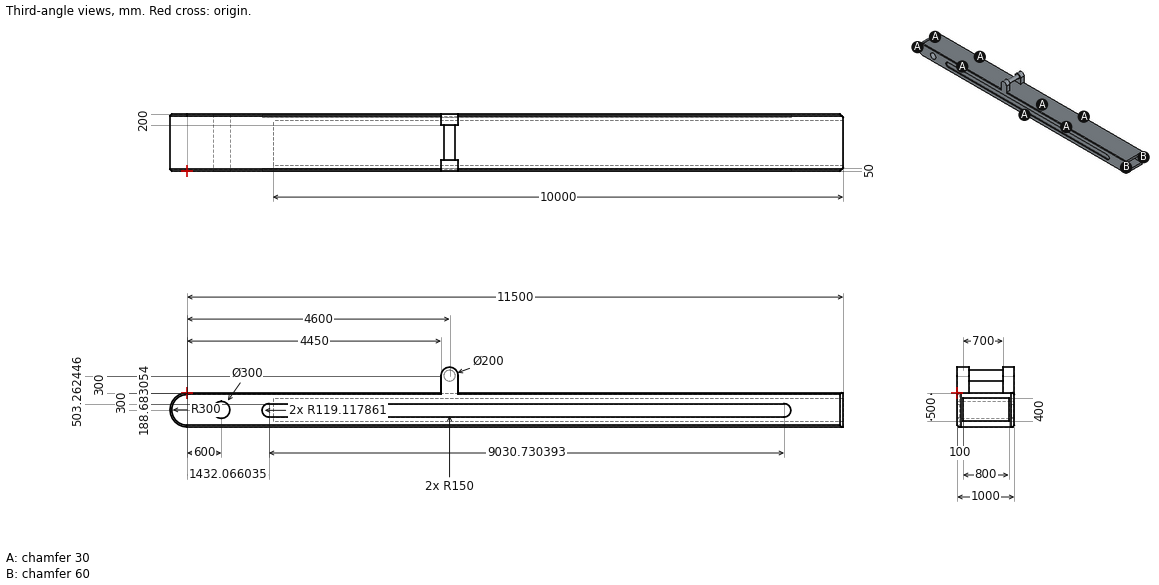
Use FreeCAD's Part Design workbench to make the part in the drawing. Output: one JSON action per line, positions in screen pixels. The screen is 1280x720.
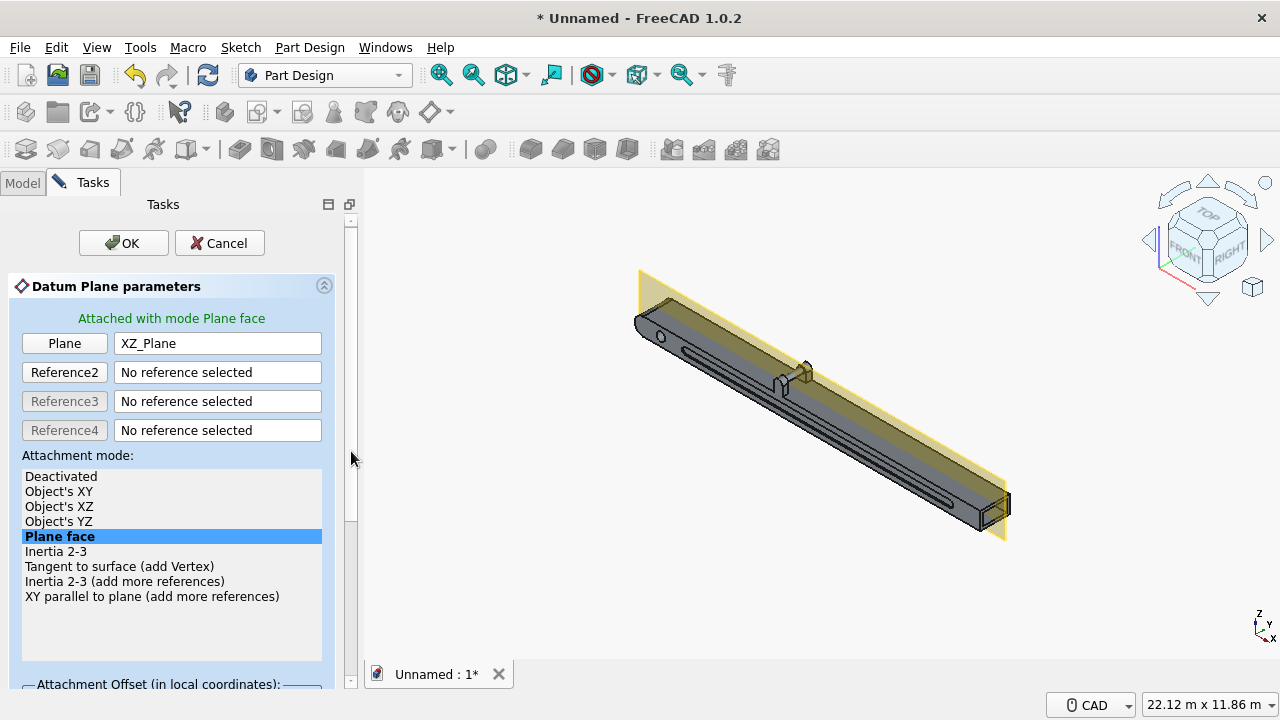
{"action": "left_click", "coordinate": [124, 243]}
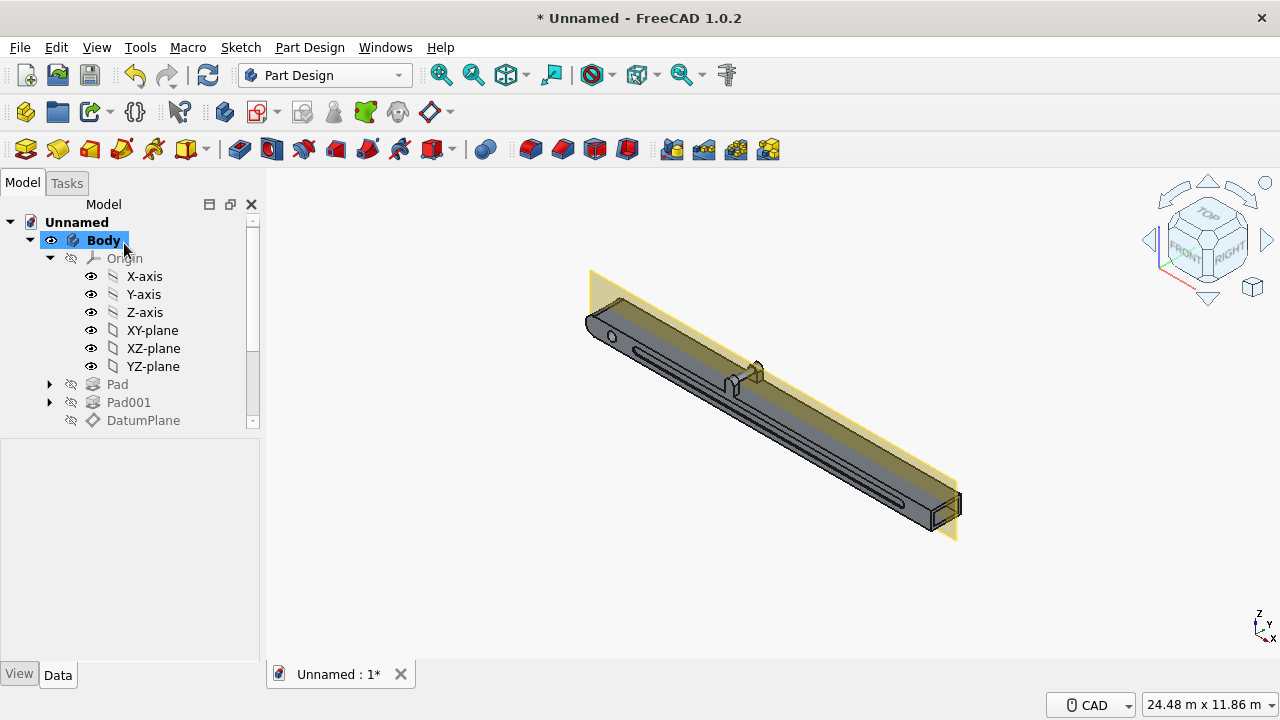
{"action": "scroll", "coordinate": [100, 326], "scroll_direction": "down", "scroll_amount": 3}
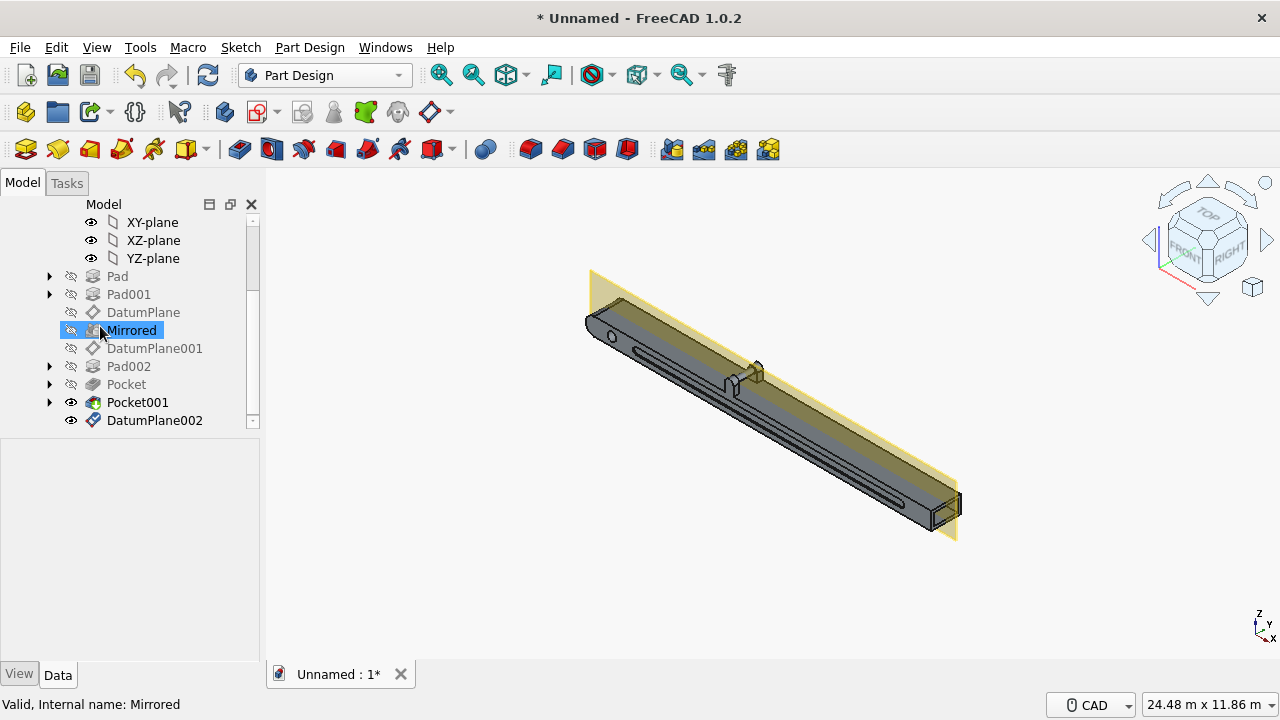
{"action": "left_click", "coordinate": [116, 402]}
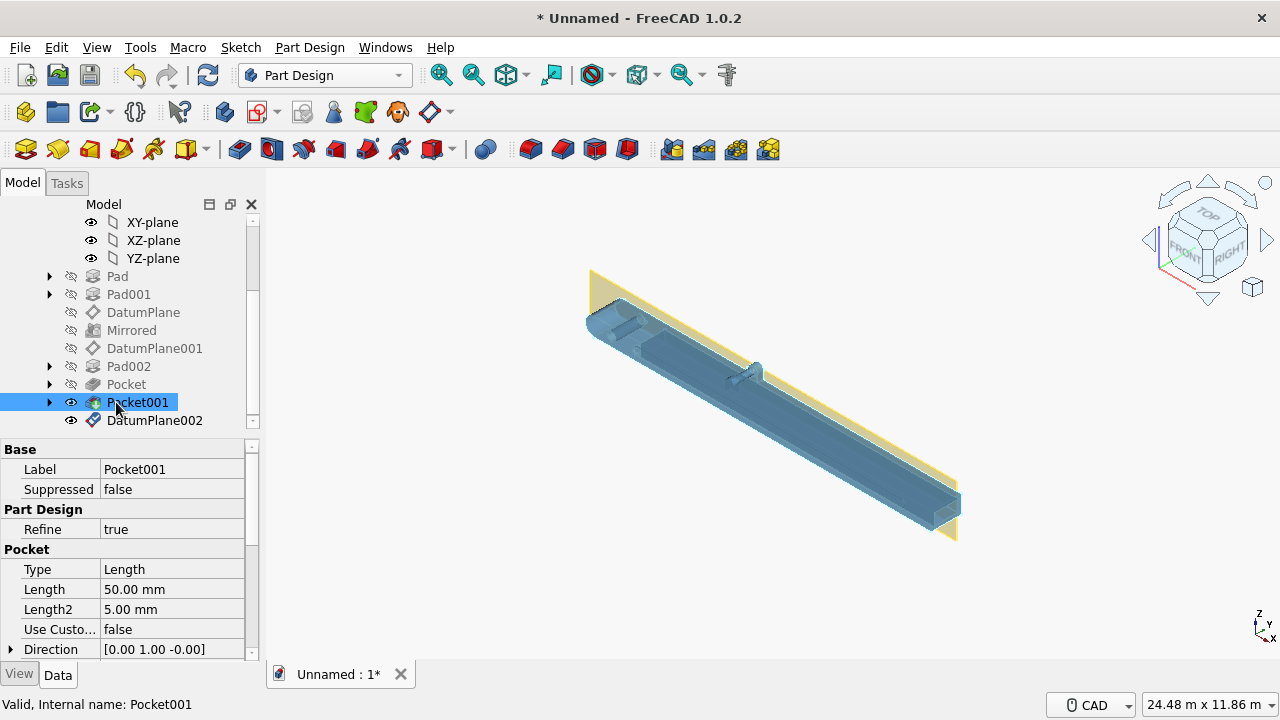
{"action": "left_click", "coordinate": [672, 150]}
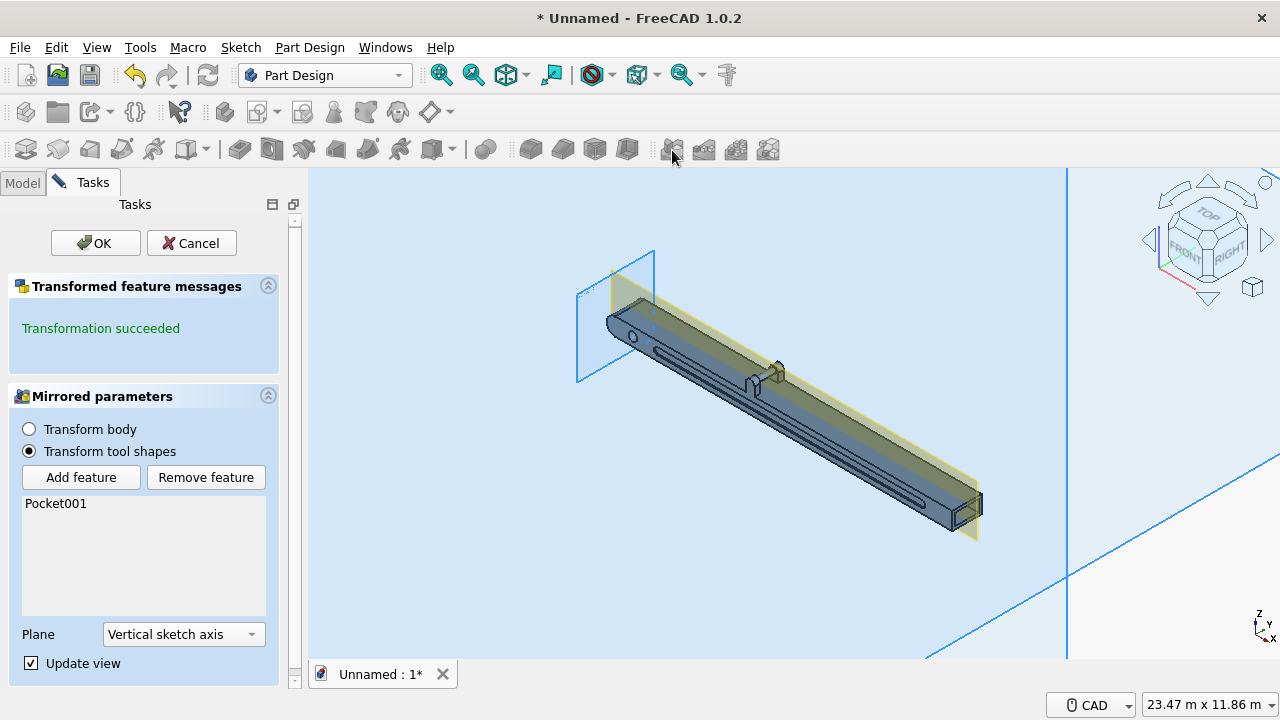
{"action": "left_click", "coordinate": [184, 634]}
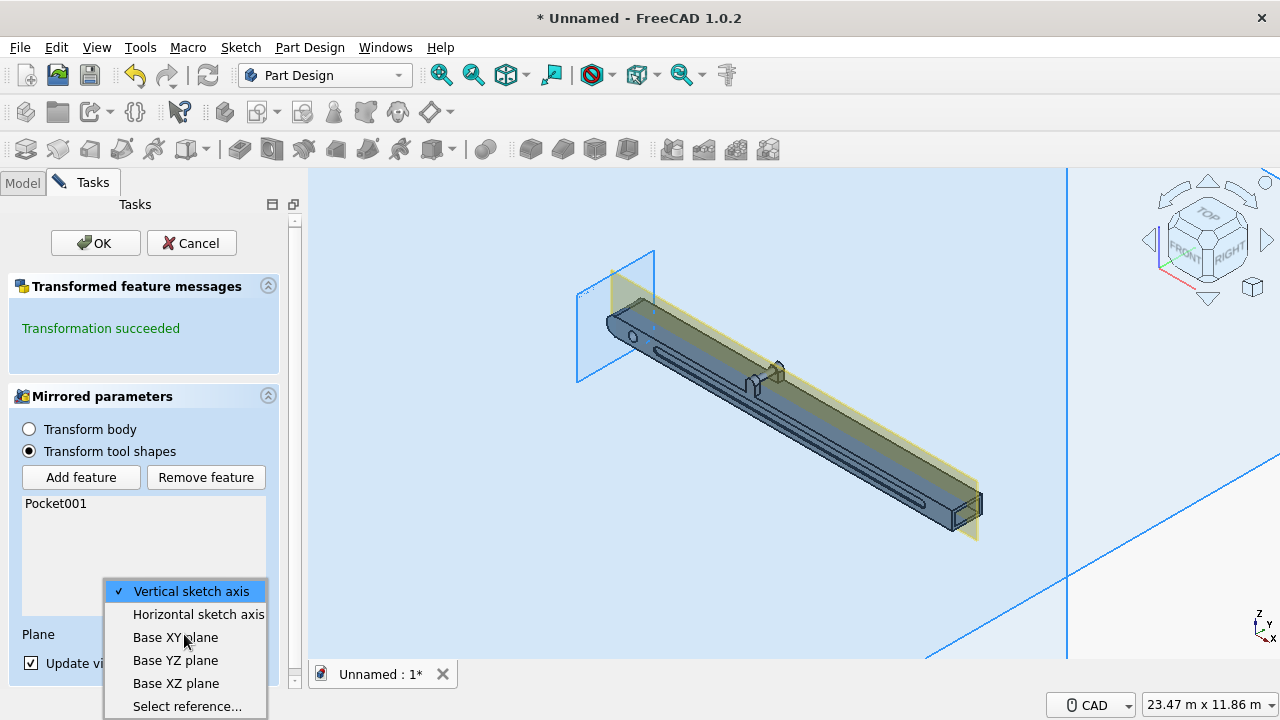
{"action": "left_click", "coordinate": [184, 706]}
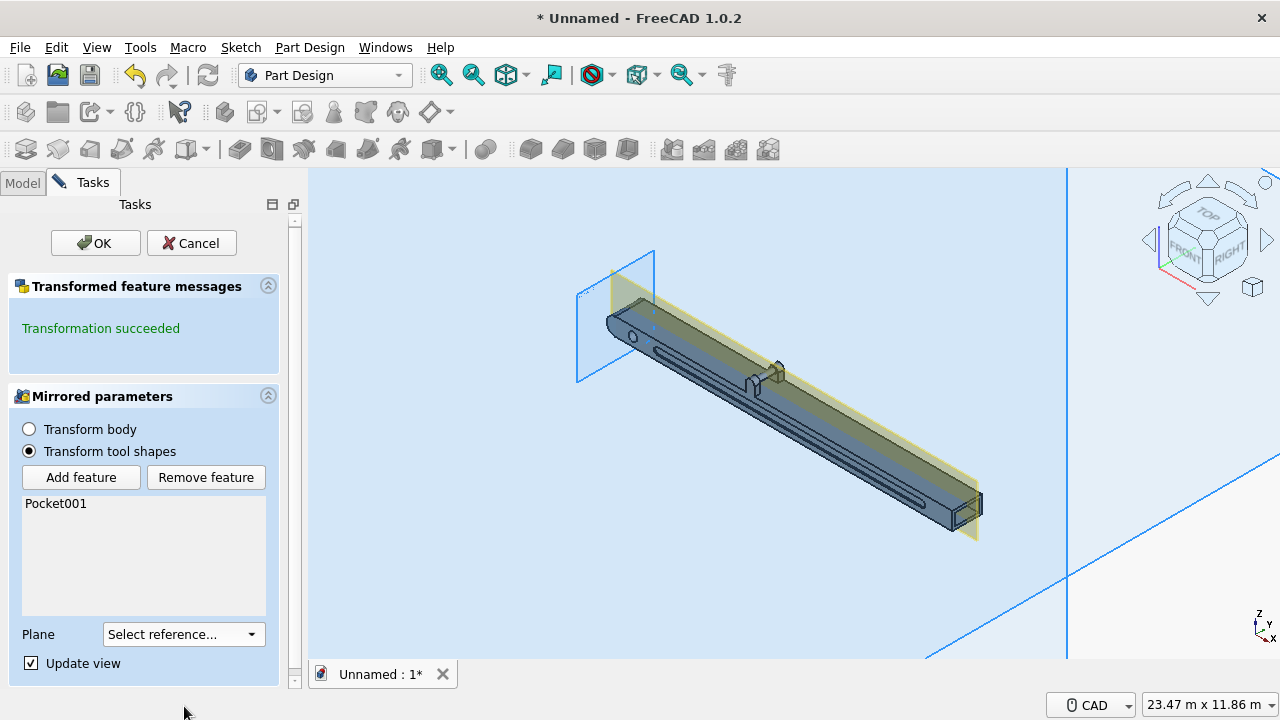
{"action": "left_click", "coordinate": [23, 182]}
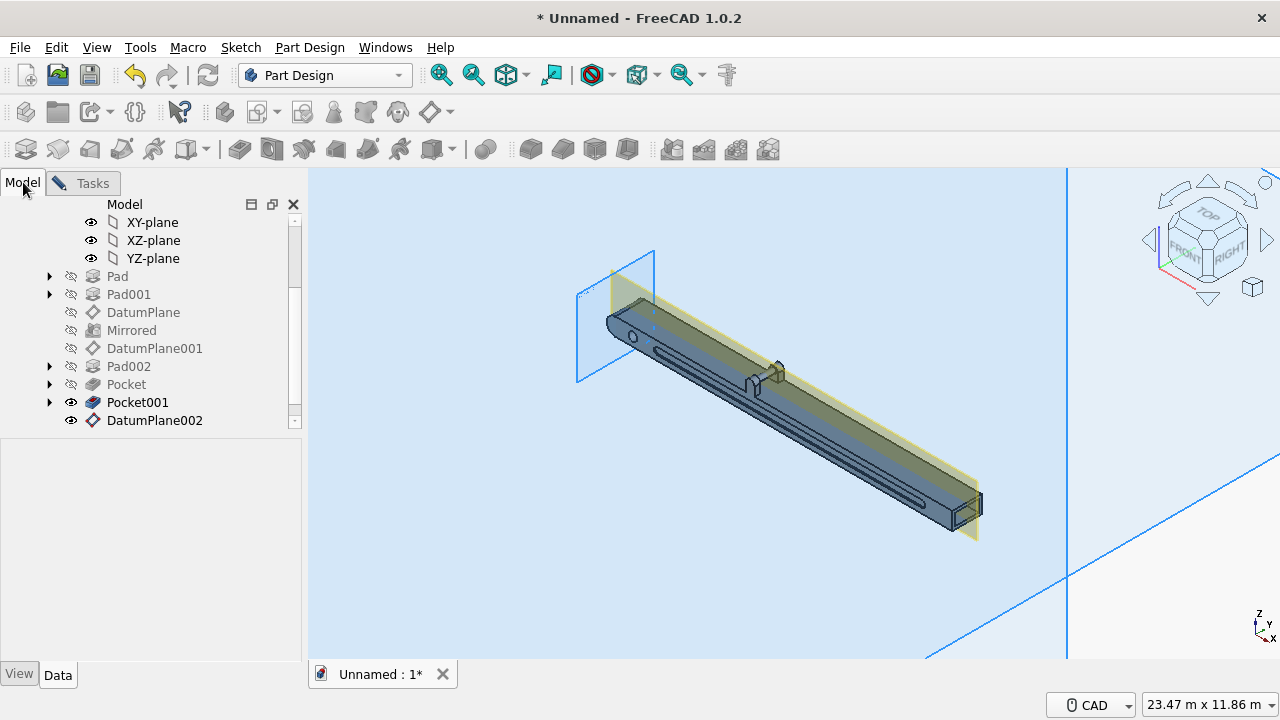
{"action": "left_click", "coordinate": [116, 420]}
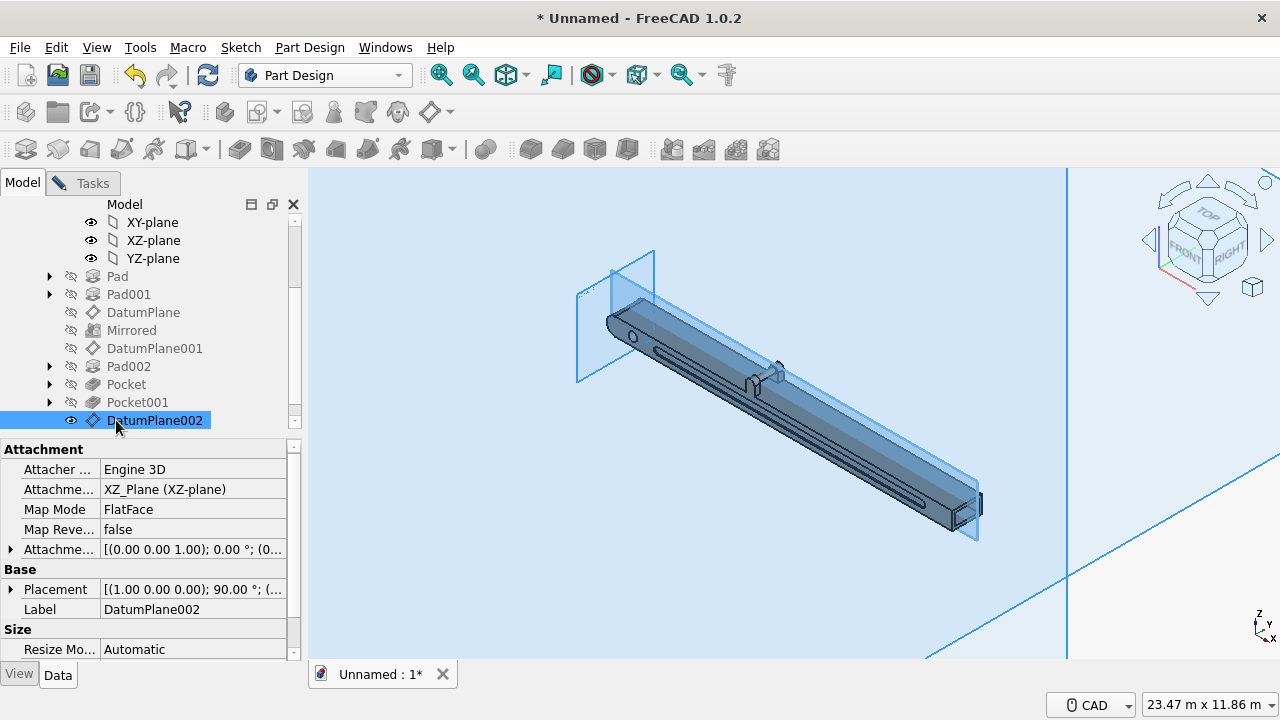
{"action": "left_click", "coordinate": [84, 182]}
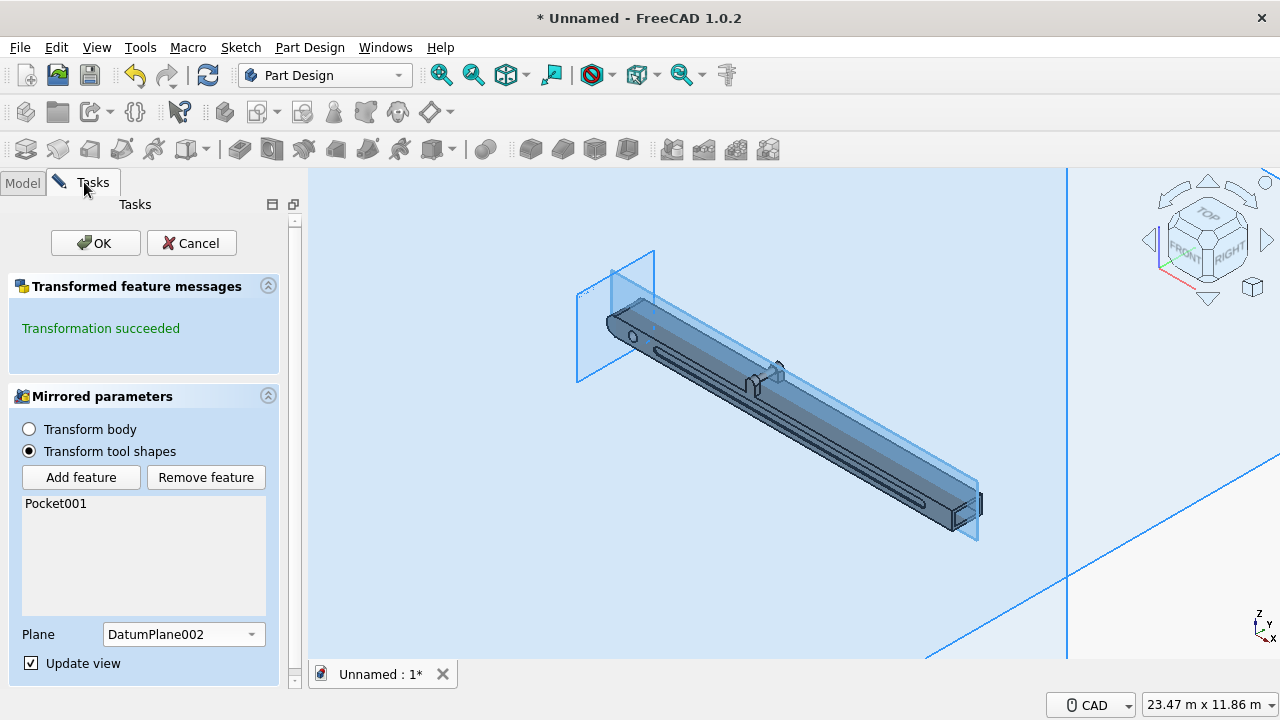
{"action": "left_click", "coordinate": [96, 243]}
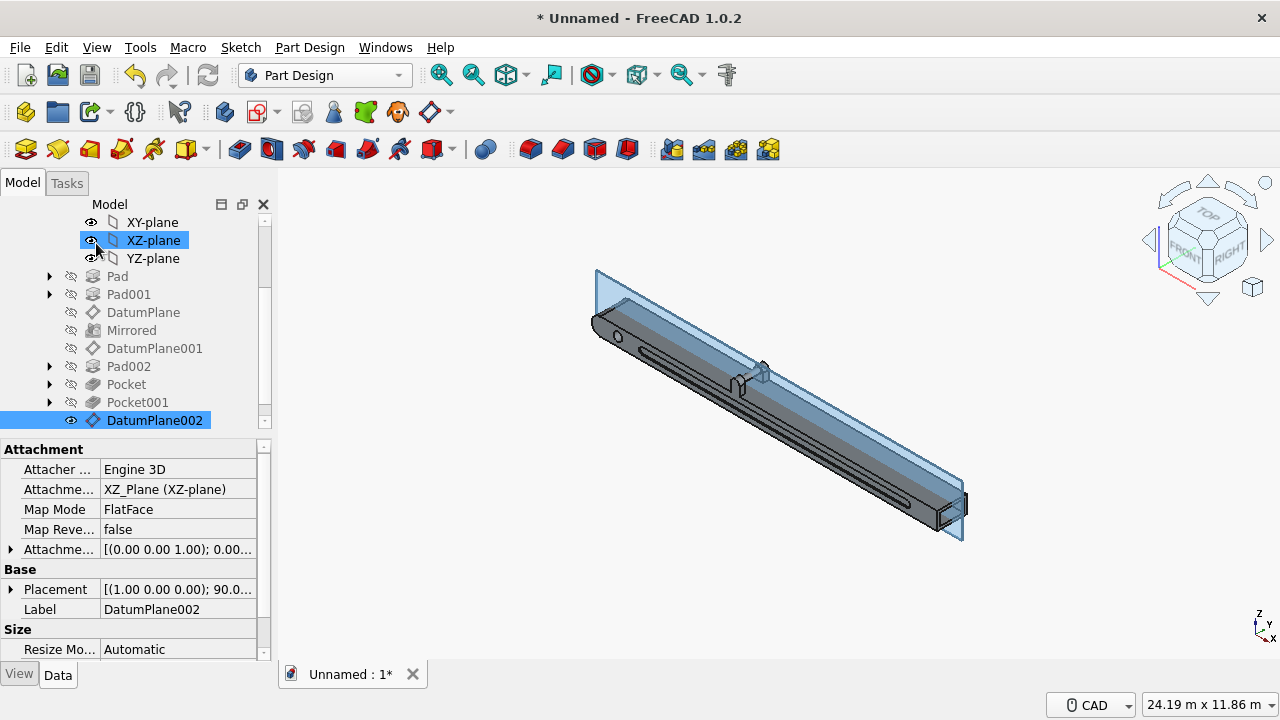
{"action": "left_click", "coordinate": [116, 420]}
{"action": "key", "text": "space"}